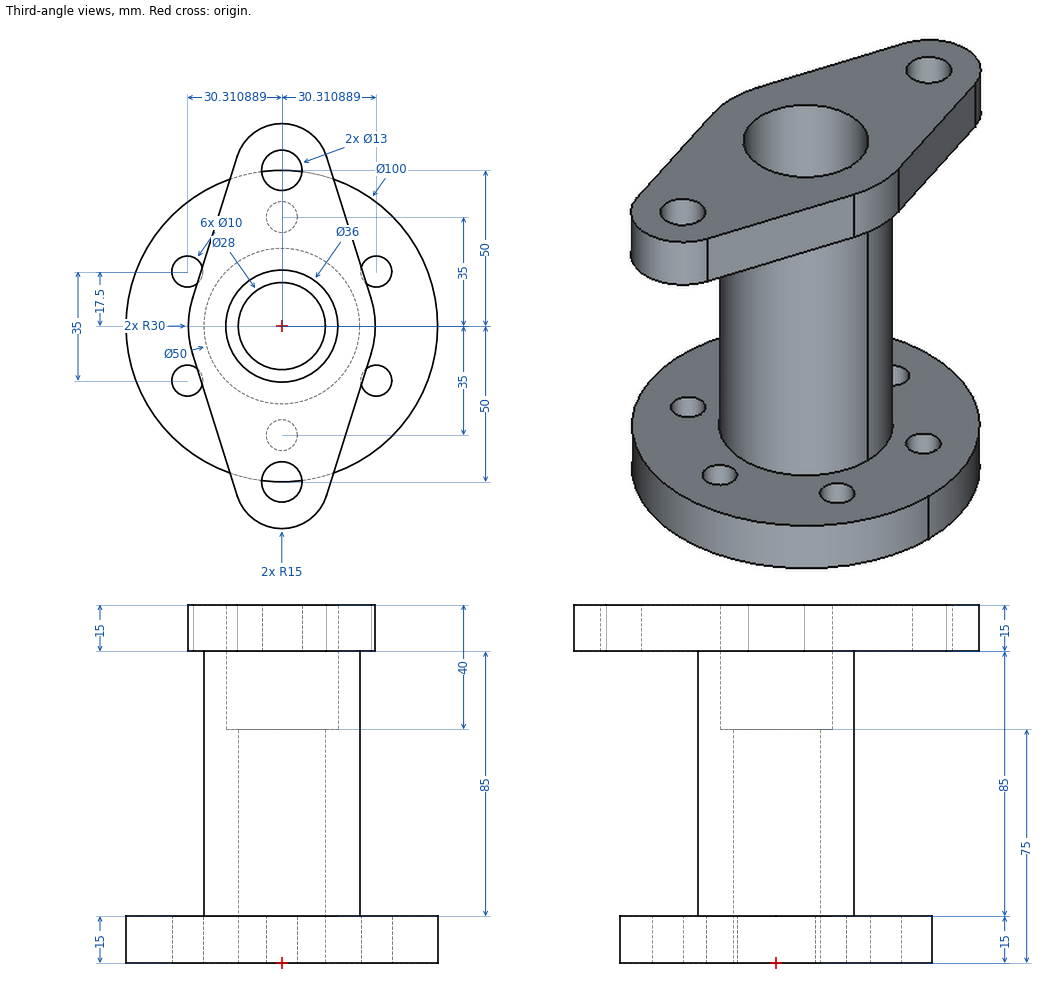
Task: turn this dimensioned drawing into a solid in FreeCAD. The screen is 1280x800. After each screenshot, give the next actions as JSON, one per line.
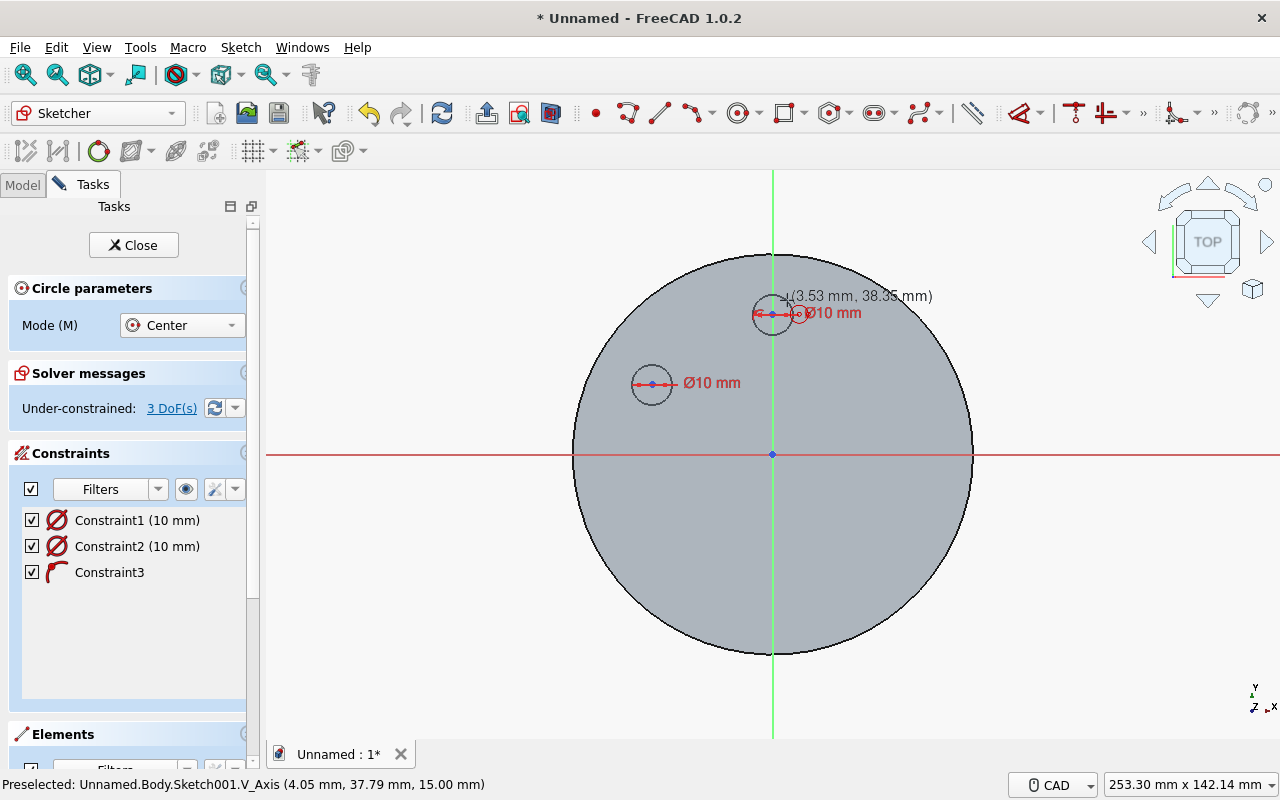
{"action": "left_click", "coordinate": [894, 384]}
{"action": "mouse_move", "coordinate": [908, 370]}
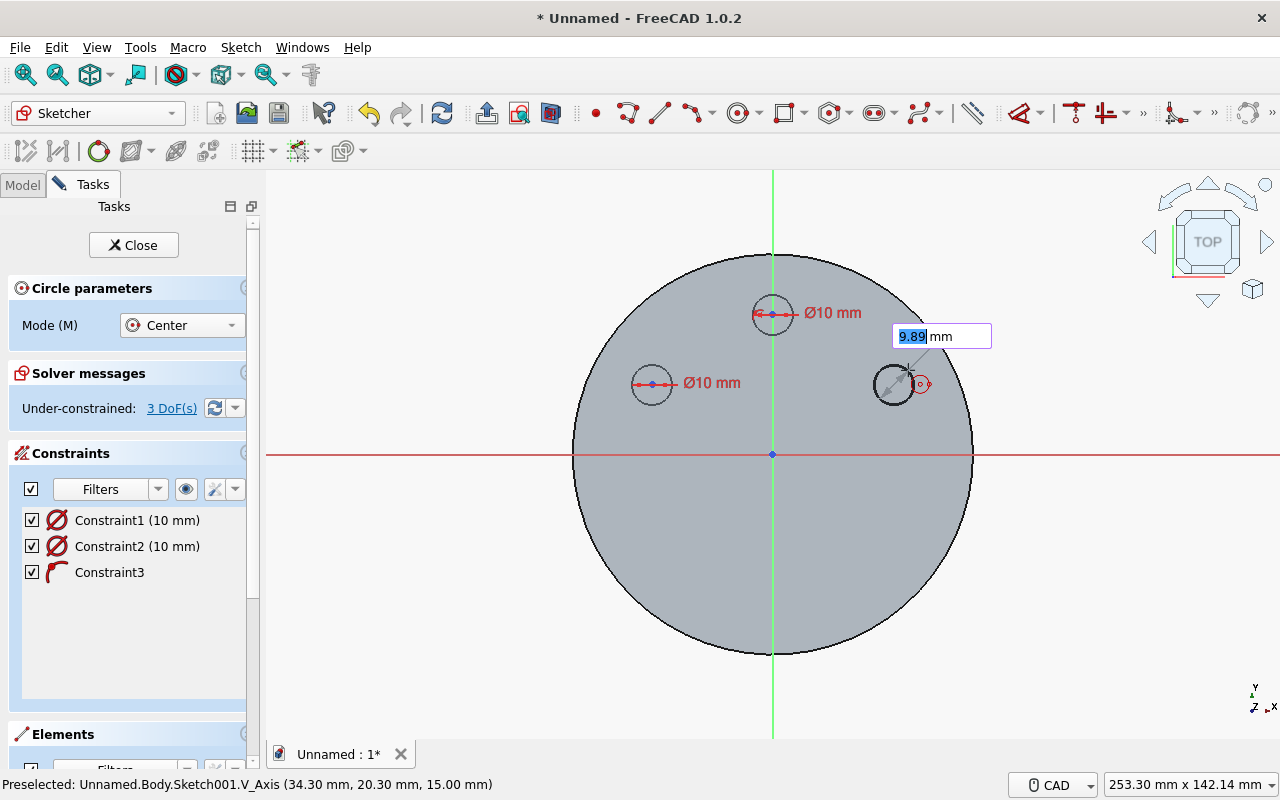
{"action": "type", "text": "10"}
{"action": "key", "text": "Return"}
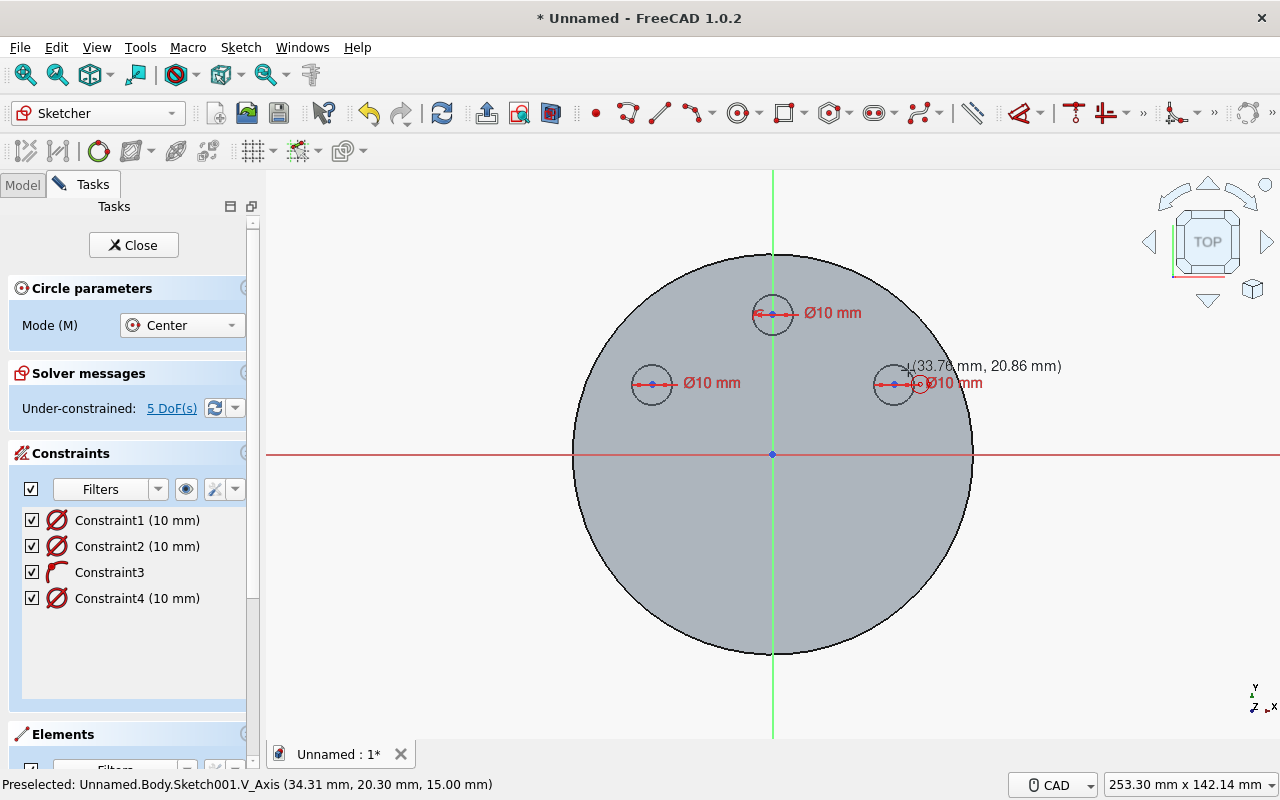
{"action": "left_click", "coordinate": [652, 525]}
{"action": "mouse_move", "coordinate": [666, 510]}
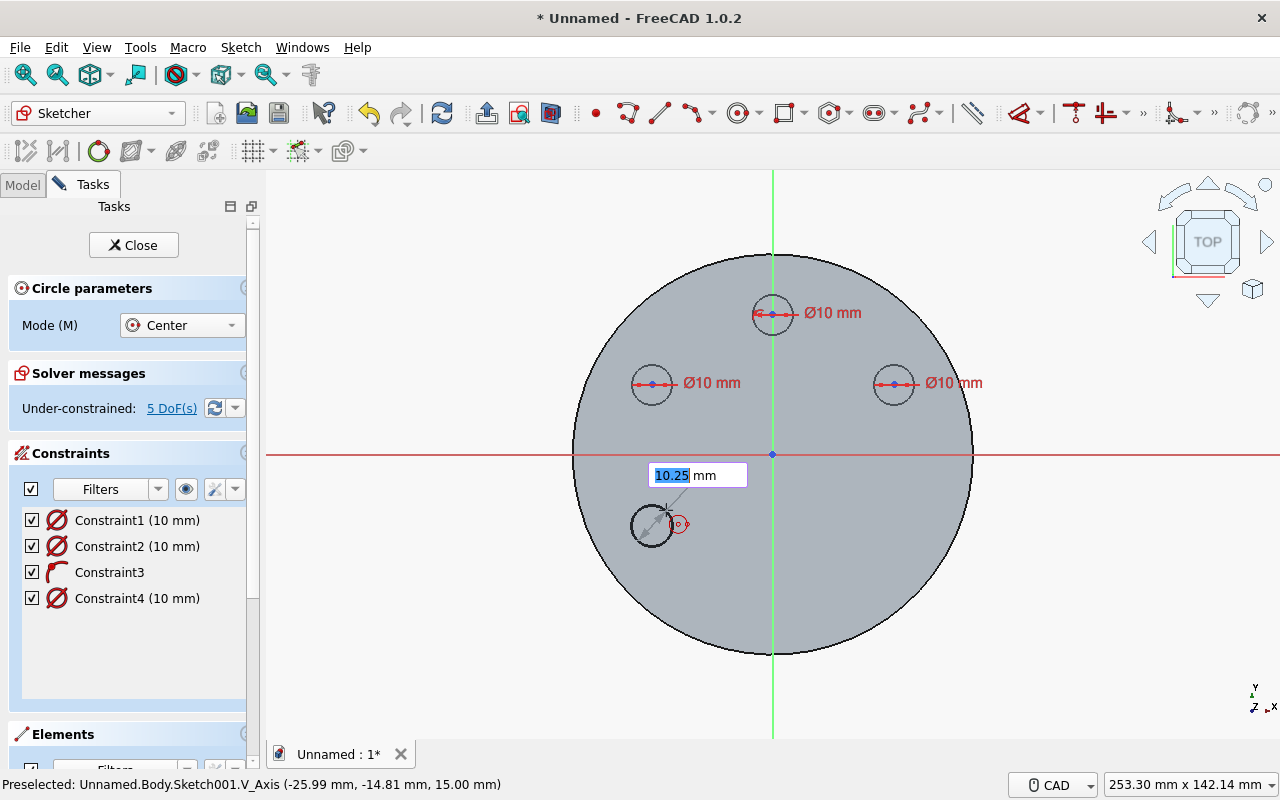
{"action": "type", "text": "10"}
{"action": "key", "text": "Return"}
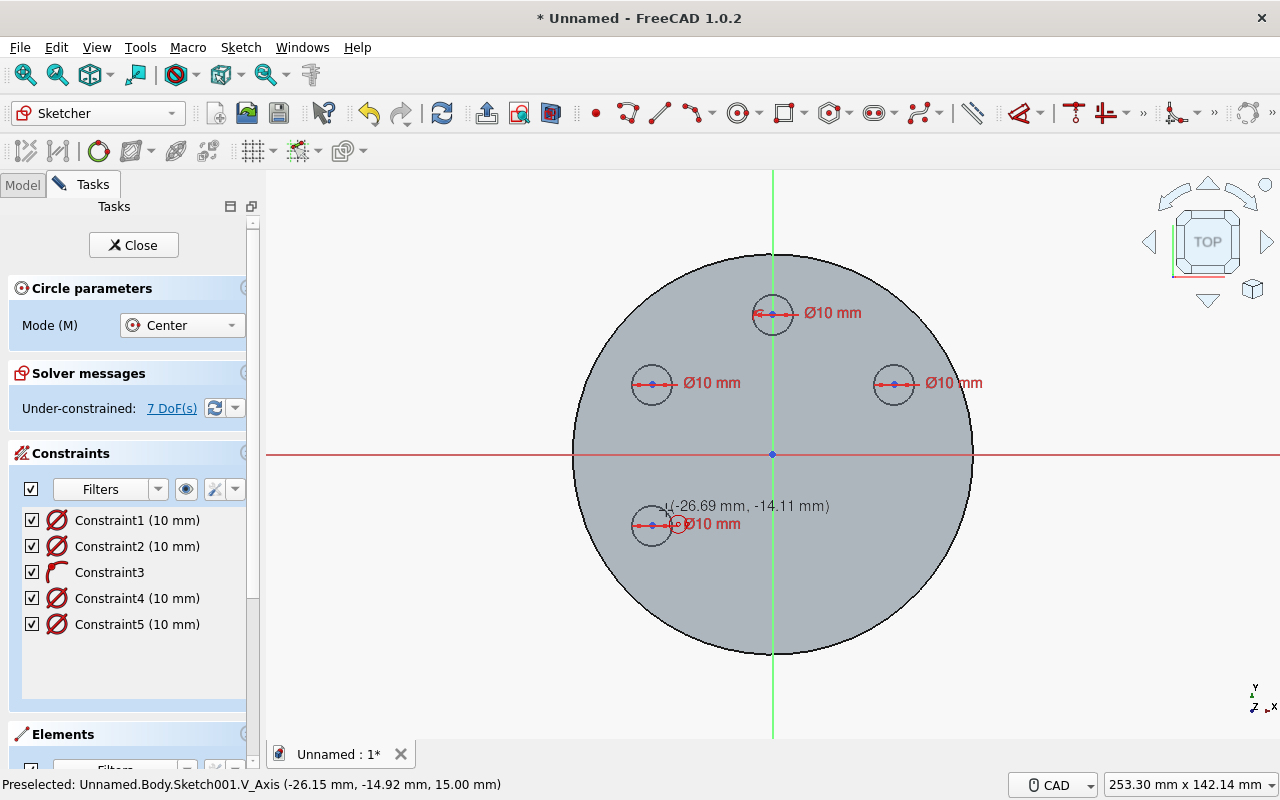
{"action": "left_click", "coordinate": [894, 525]}
{"action": "mouse_move", "coordinate": [908, 510]}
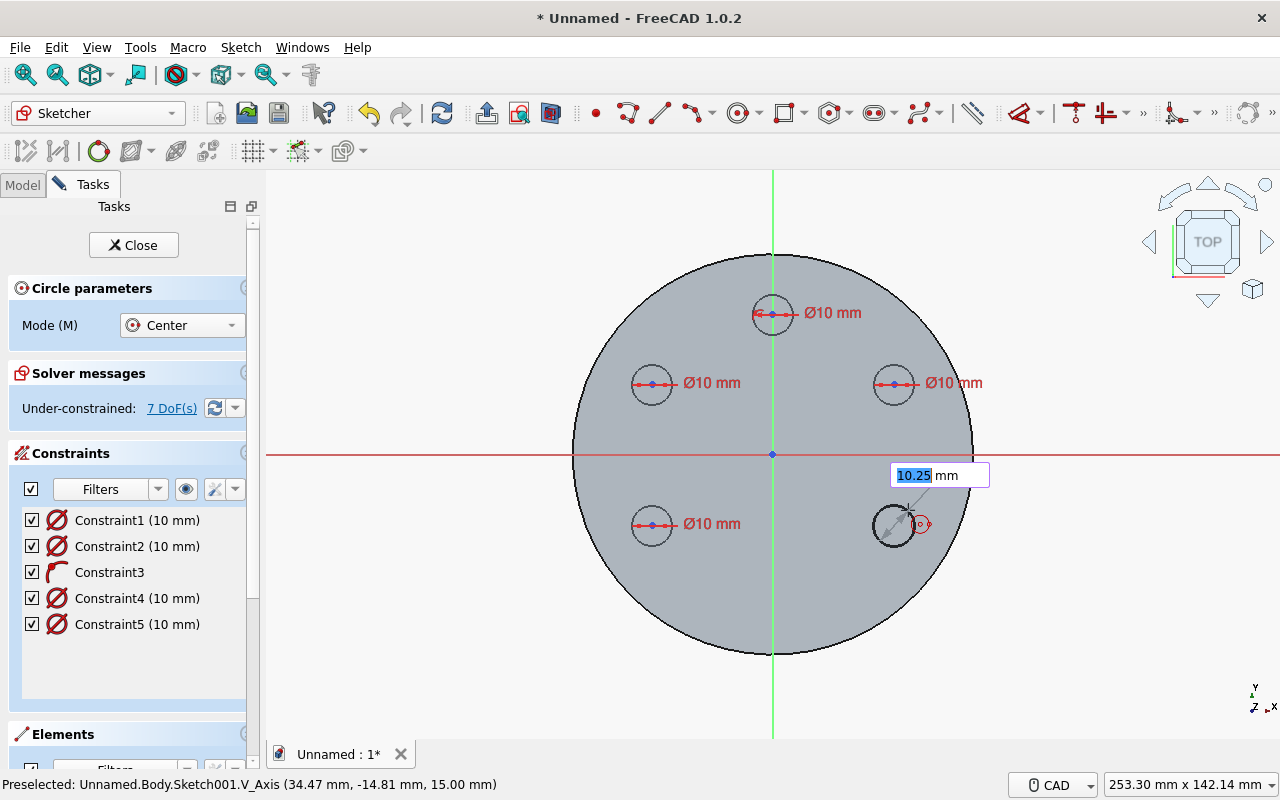
{"action": "type", "text": "10"}
{"action": "key", "text": "Return"}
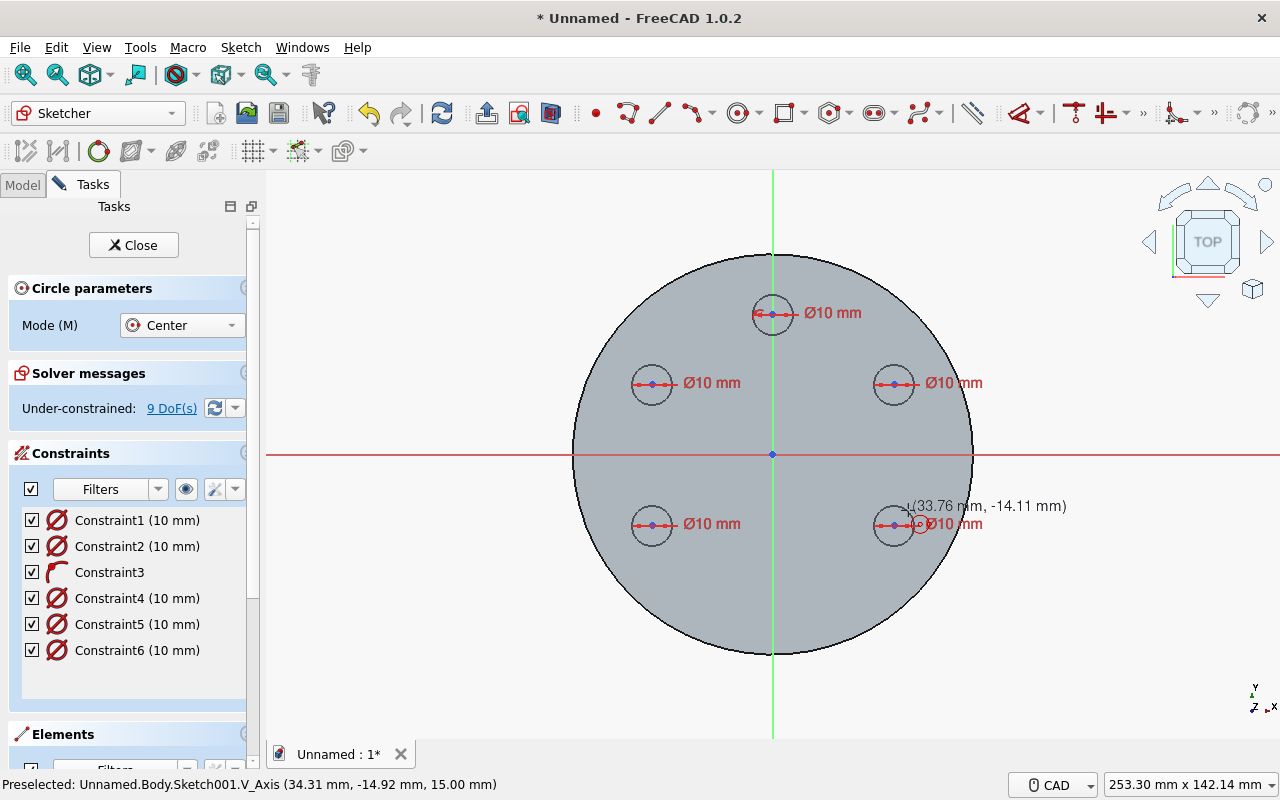
{"action": "left_click", "coordinate": [773, 595]}
{"action": "mouse_move", "coordinate": [787, 580]}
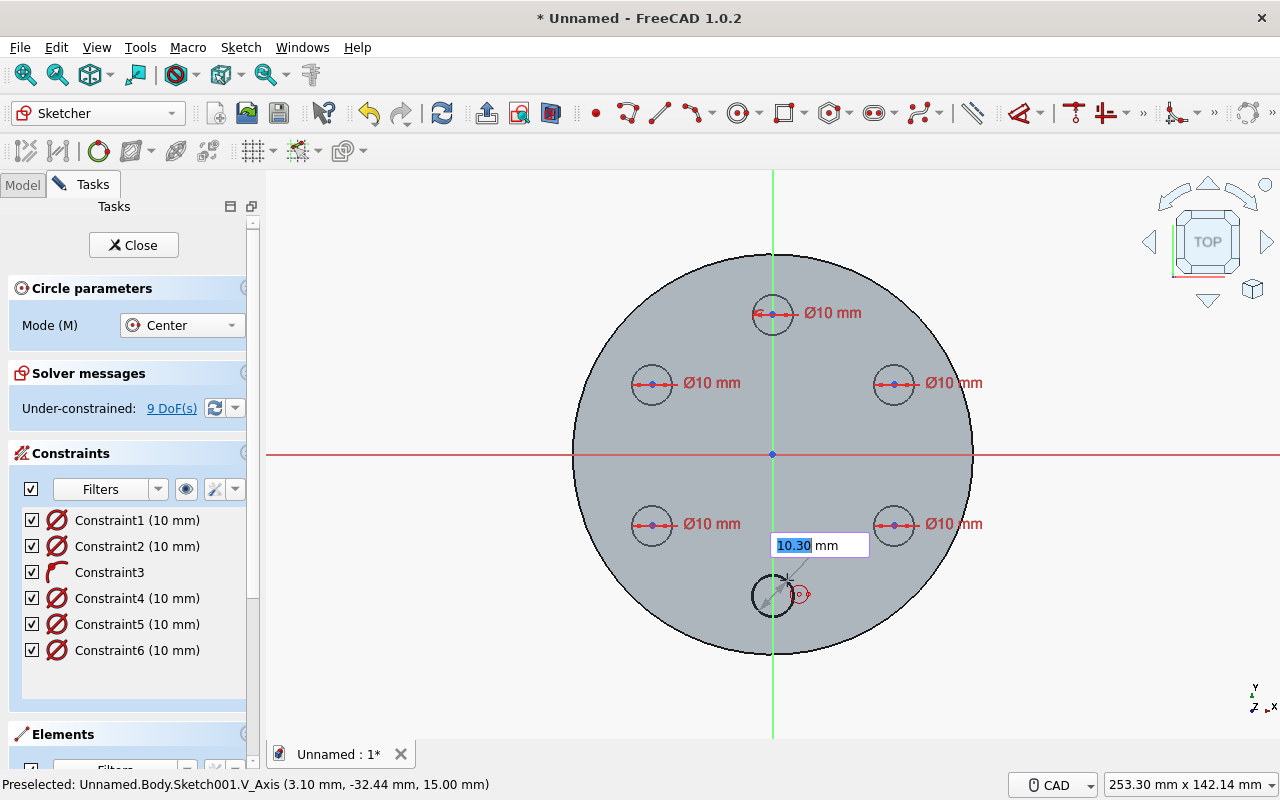
{"action": "type", "text": "10"}
{"action": "key", "text": "Return"}
{"action": "key", "text": "Escape"}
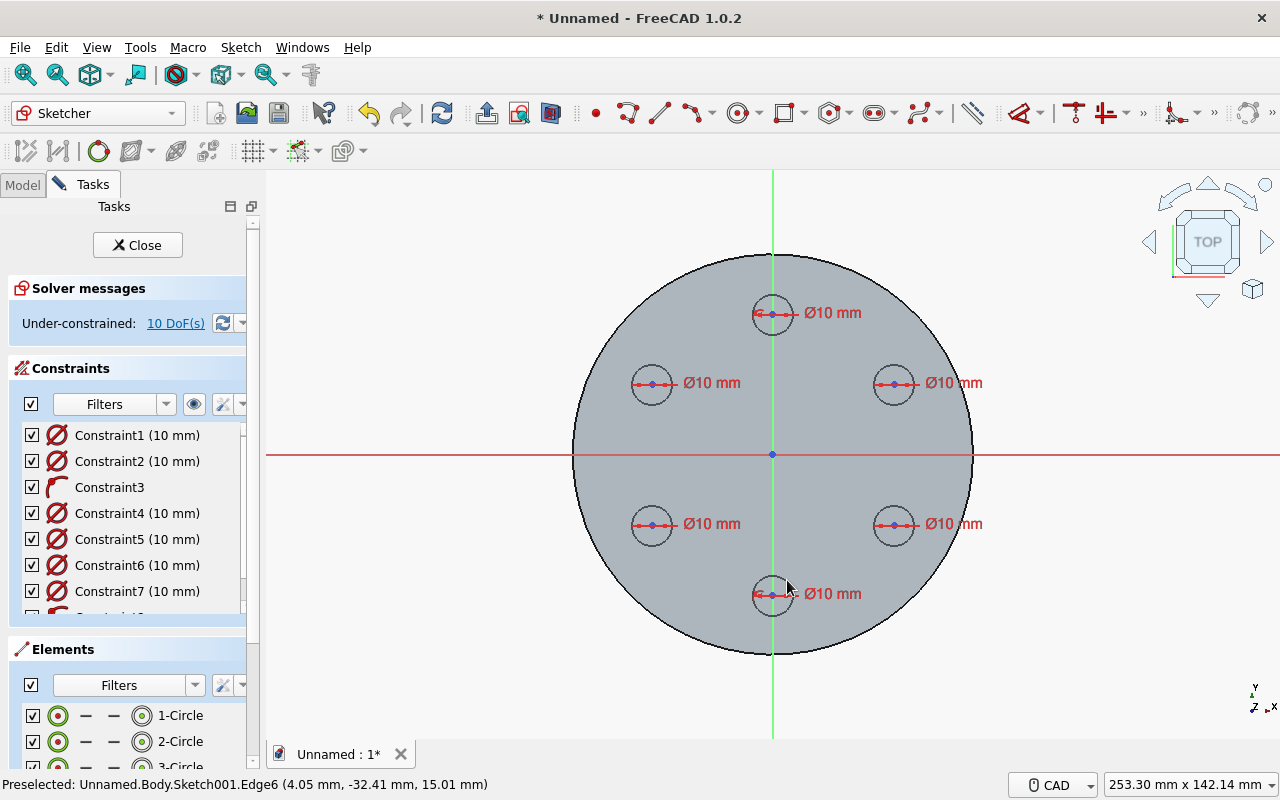
{"action": "left_click", "coordinate": [652, 385]}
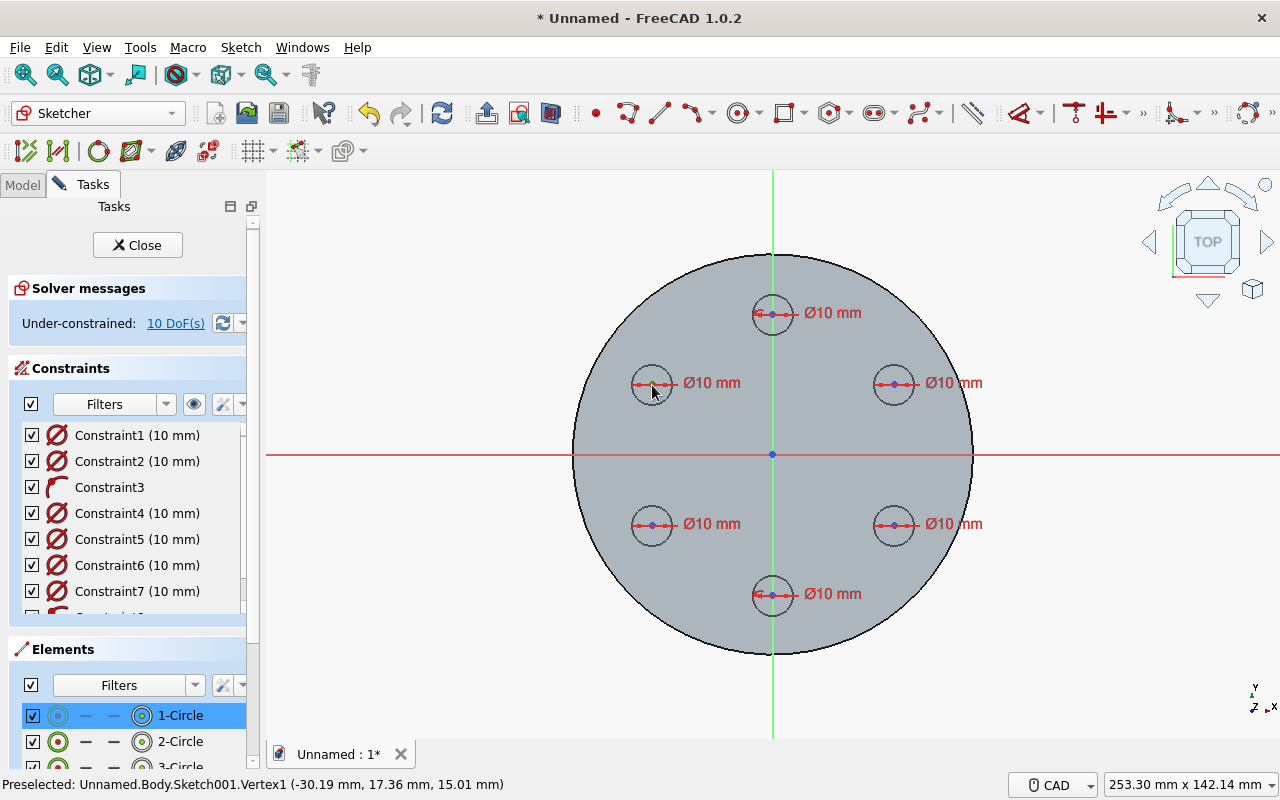
{"action": "left_click", "coordinate": [894, 385]}